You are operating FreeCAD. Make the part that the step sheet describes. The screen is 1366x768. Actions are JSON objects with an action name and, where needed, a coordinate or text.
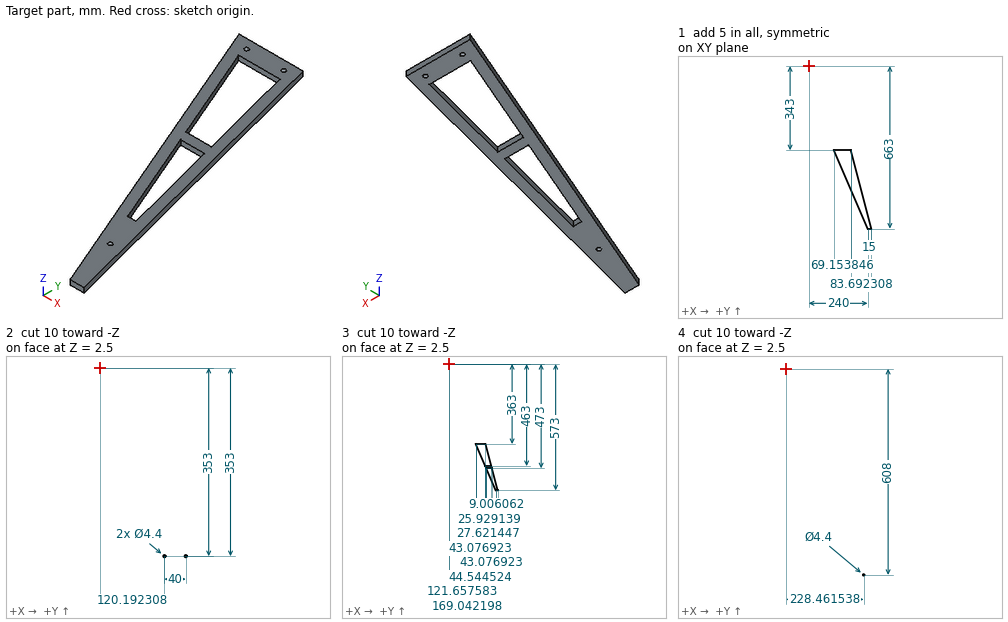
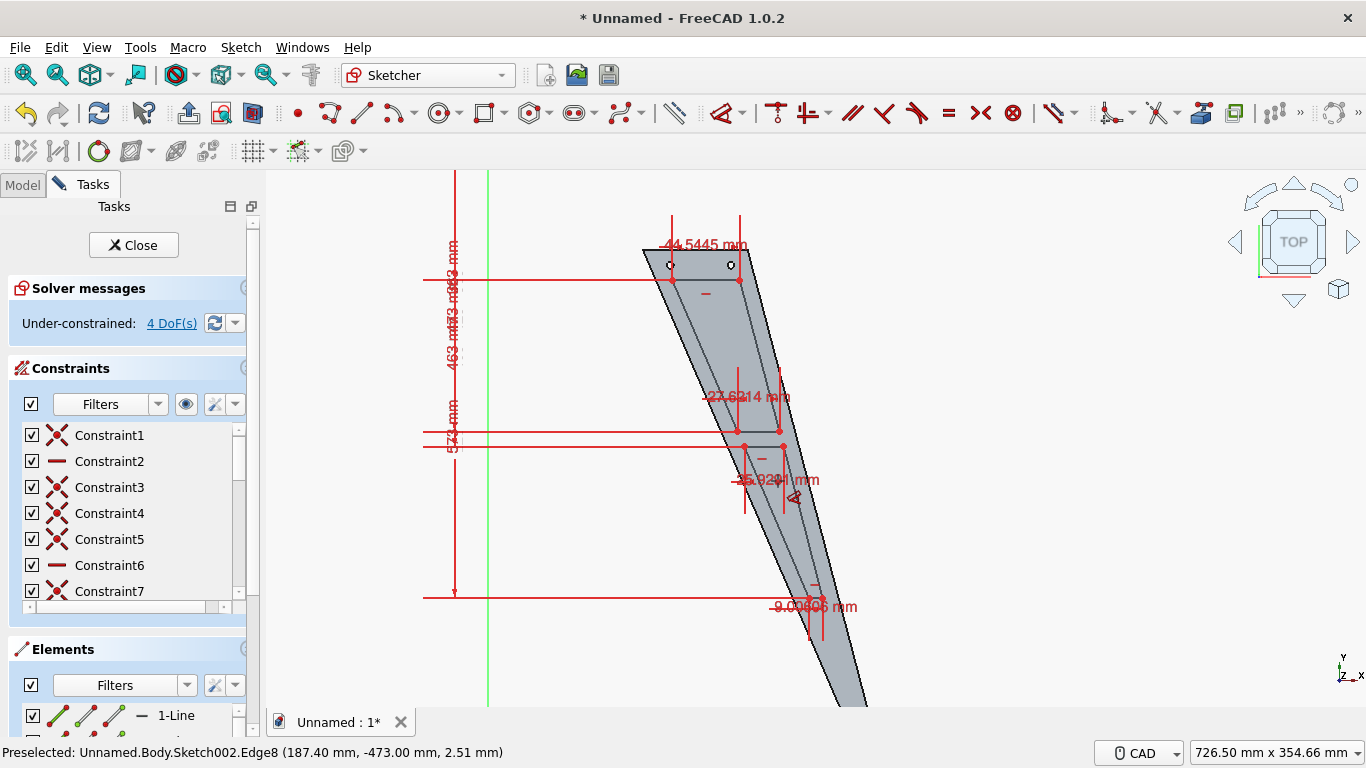
{"action": "left_click", "coordinate": [692, 326]}
{"action": "left_click", "coordinate": [705, 466]}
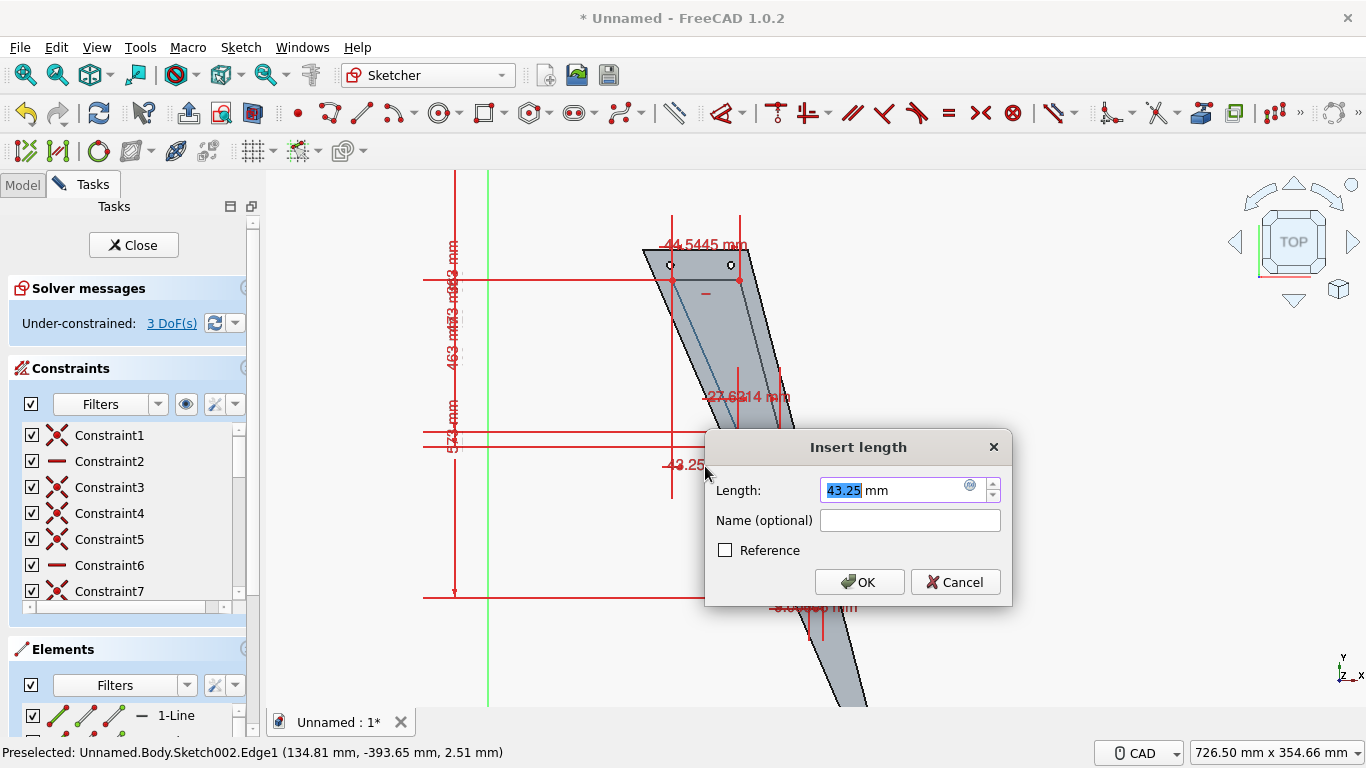
{"action": "type", "text": "43.076923"}
{"action": "key", "text": "Return"}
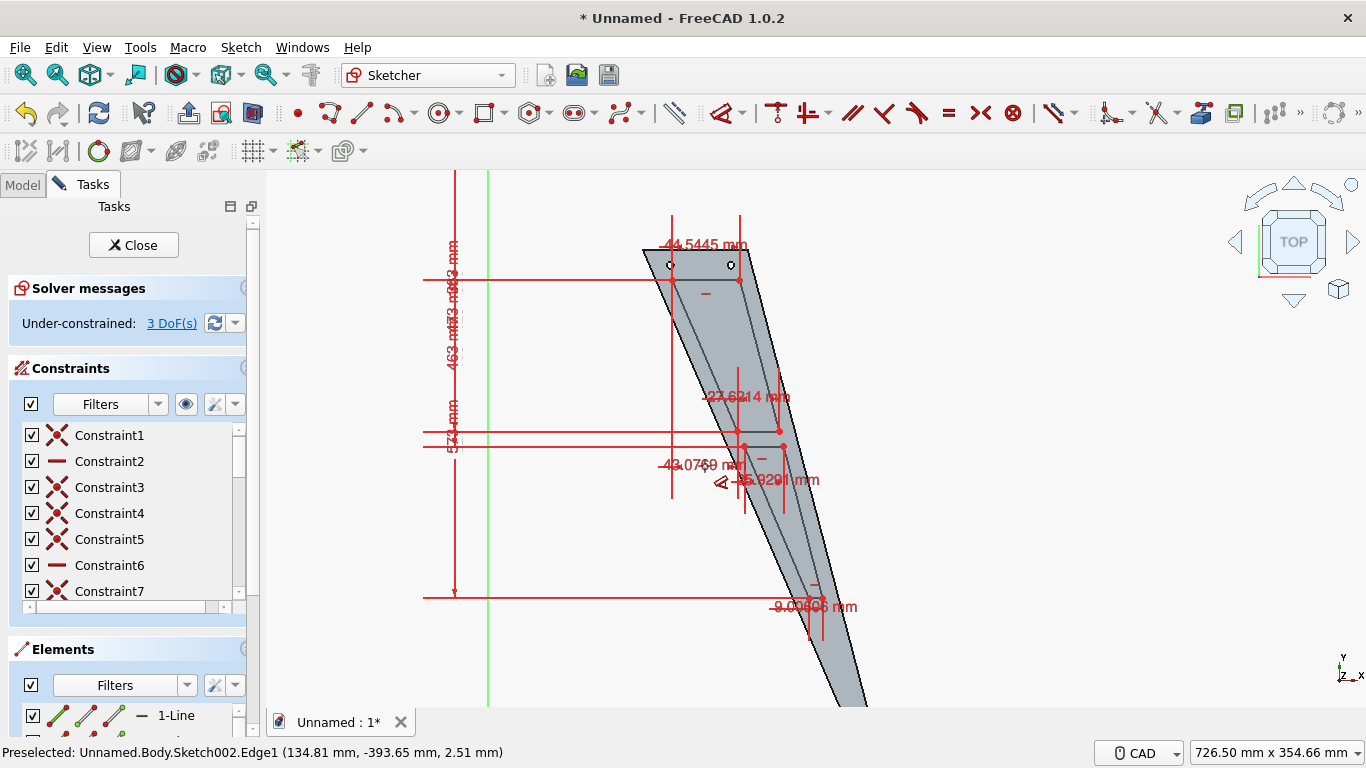
{"action": "left_click", "coordinate": [764, 492]}
{"action": "left_click", "coordinate": [777, 632]}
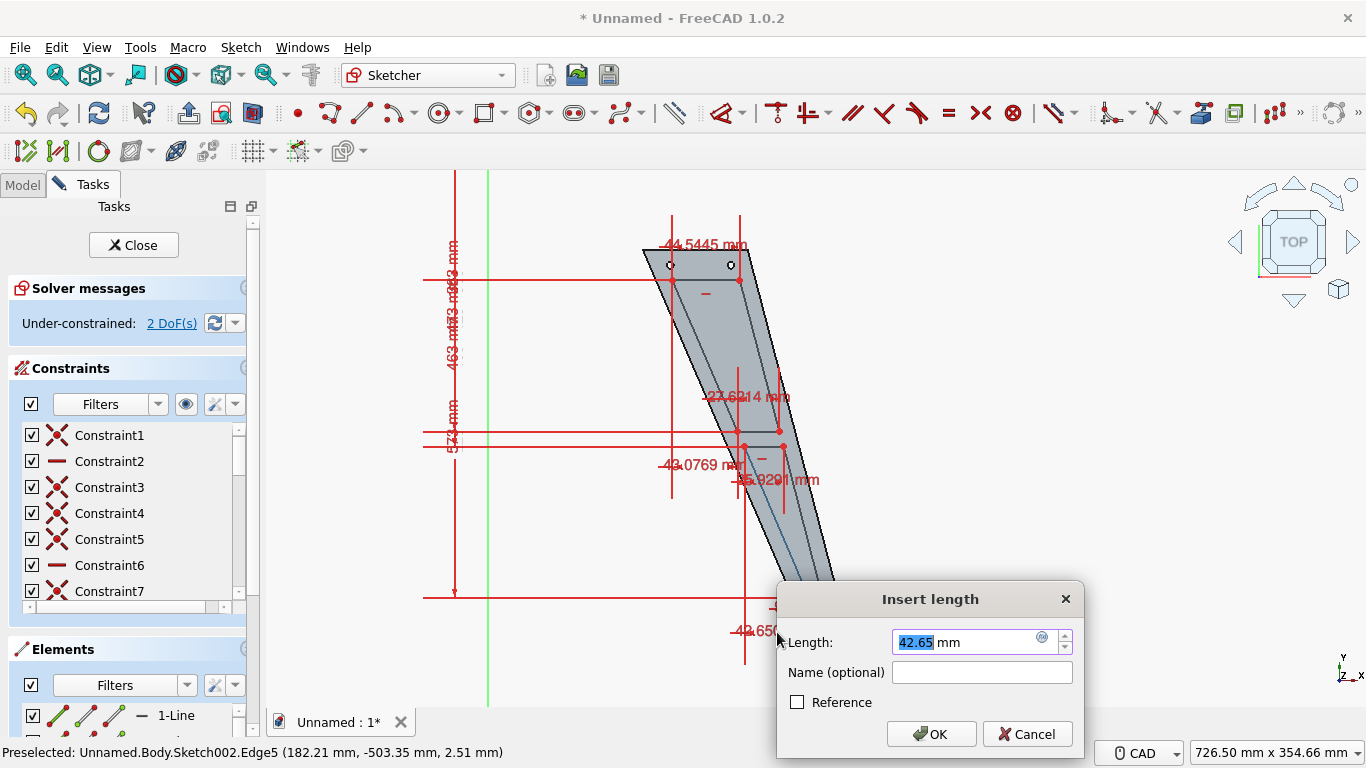
{"action": "type", "text": "43.076923"}
{"action": "key", "text": "Return"}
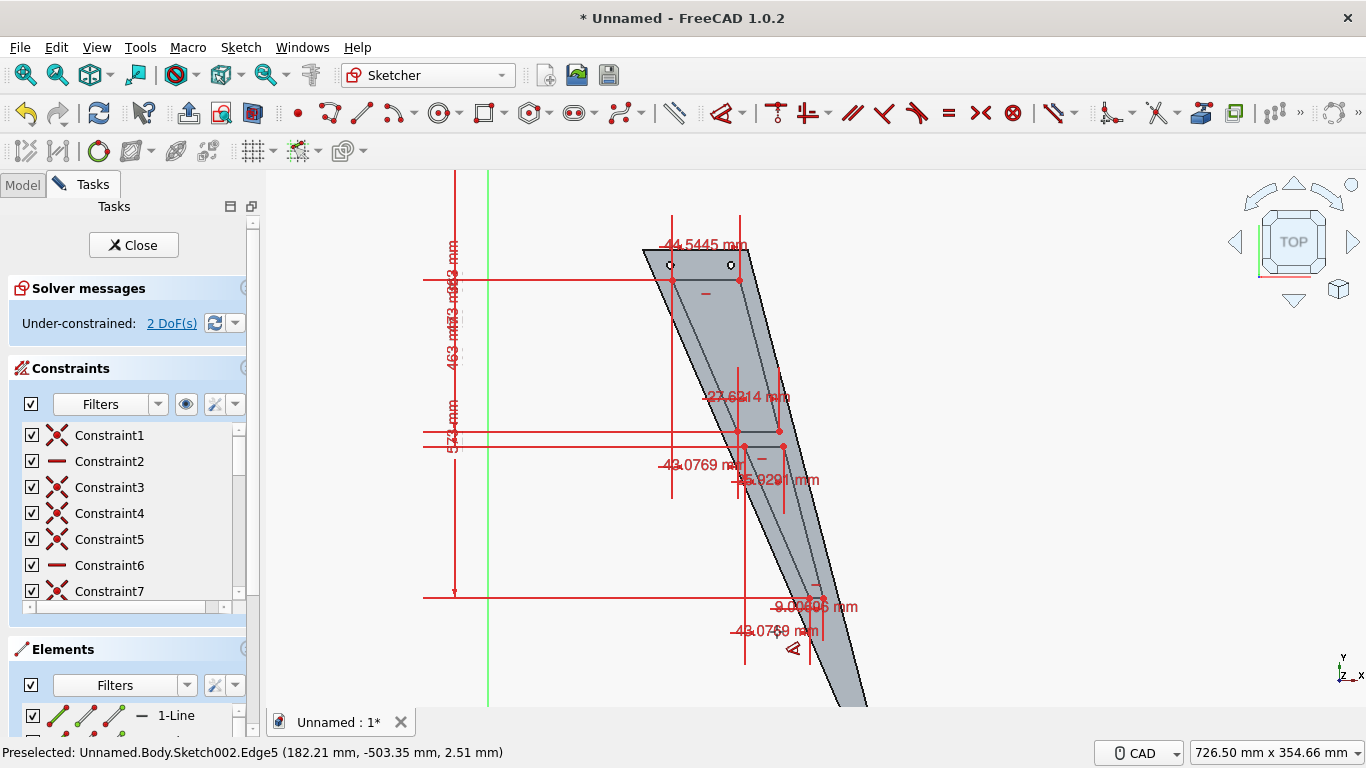
{"action": "left_click", "coordinate": [672, 280]}
{"action": "left_click", "coordinate": [580, 314]}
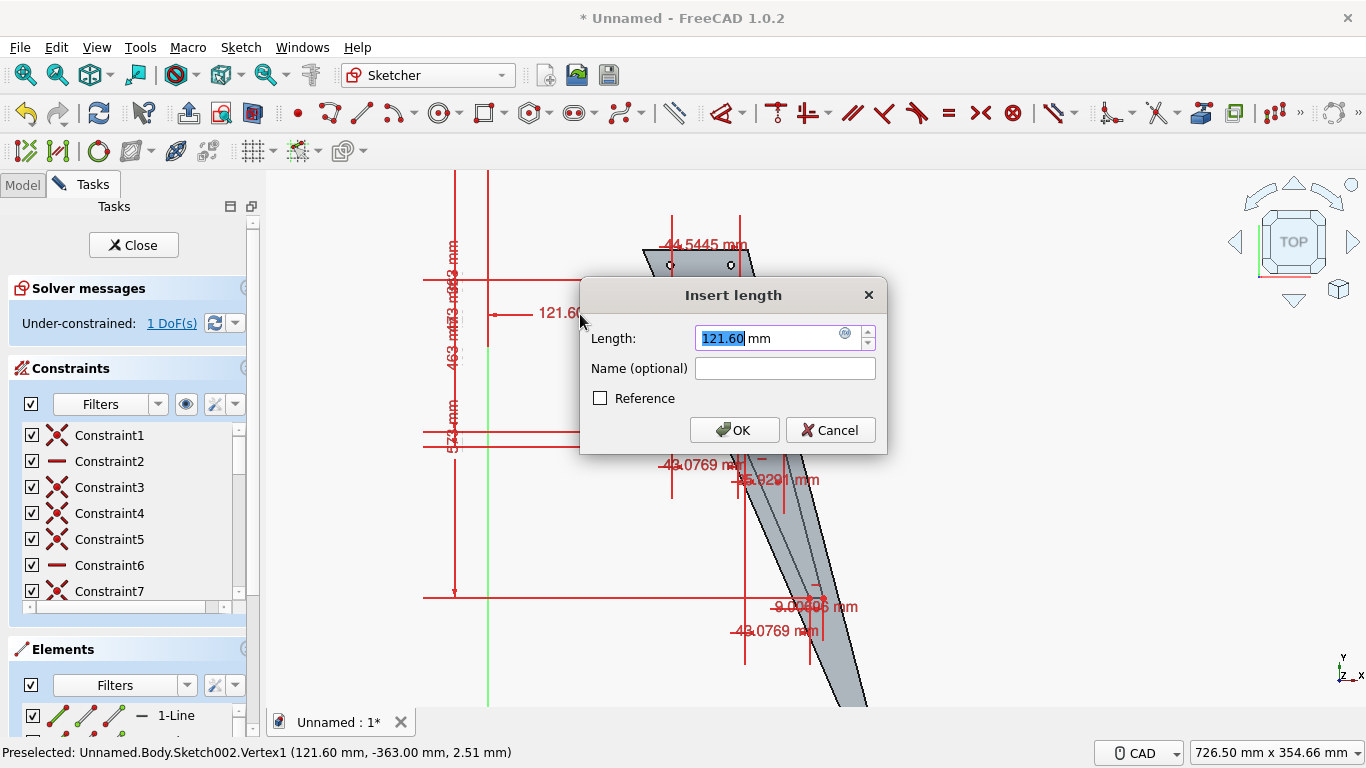
{"action": "type", "text": "121.657583"}
{"action": "key", "text": "Return"}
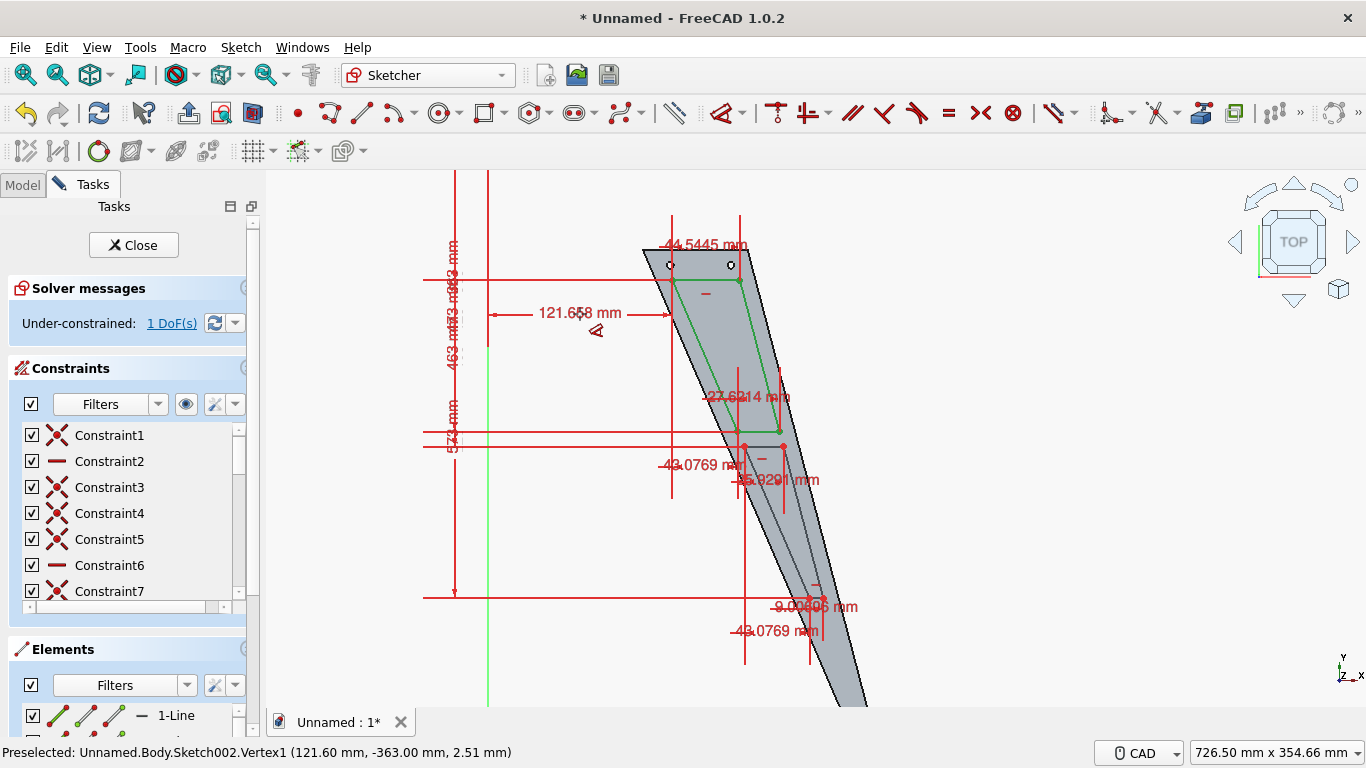
{"action": "left_click", "coordinate": [745, 447]}
{"action": "left_click", "coordinate": [616, 481]}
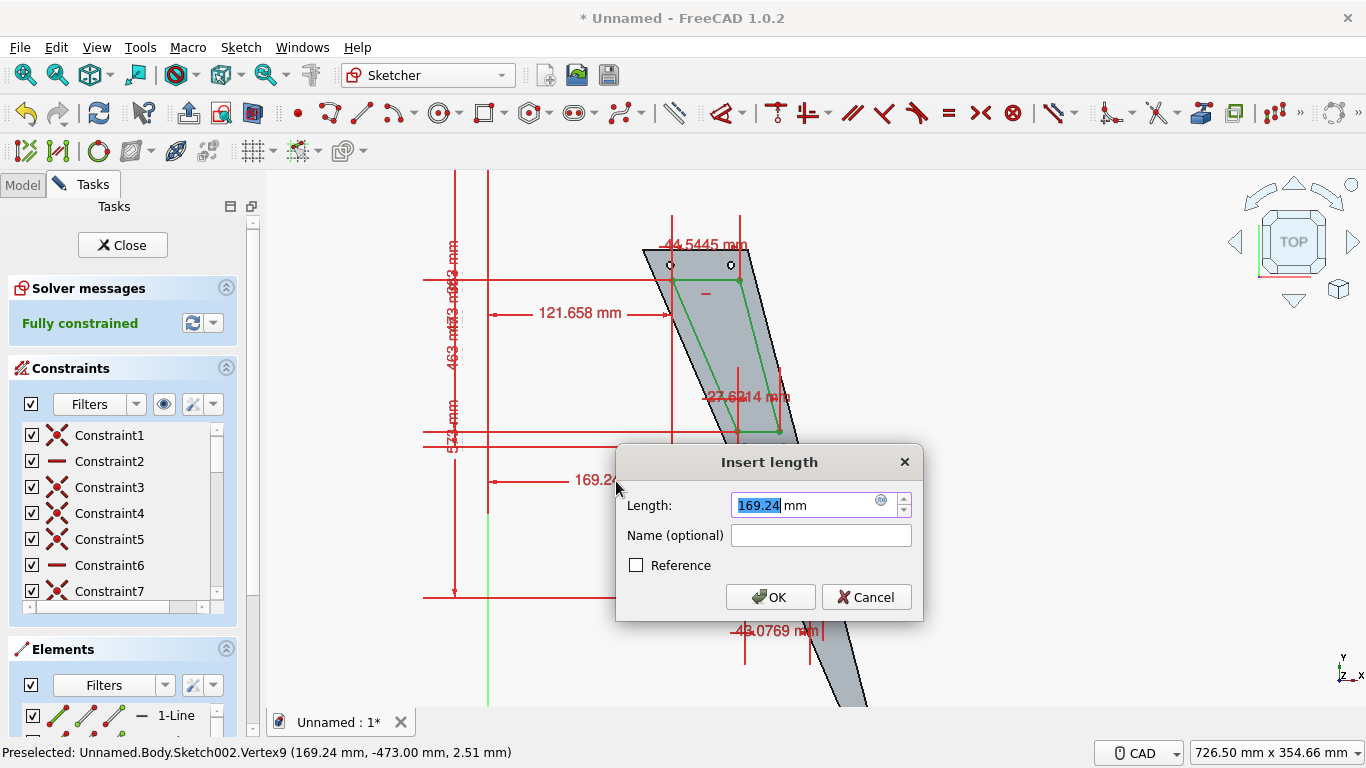
{"action": "type", "text": "169.042198"}
{"action": "key", "text": "Return"}
{"action": "key", "text": "Escape"}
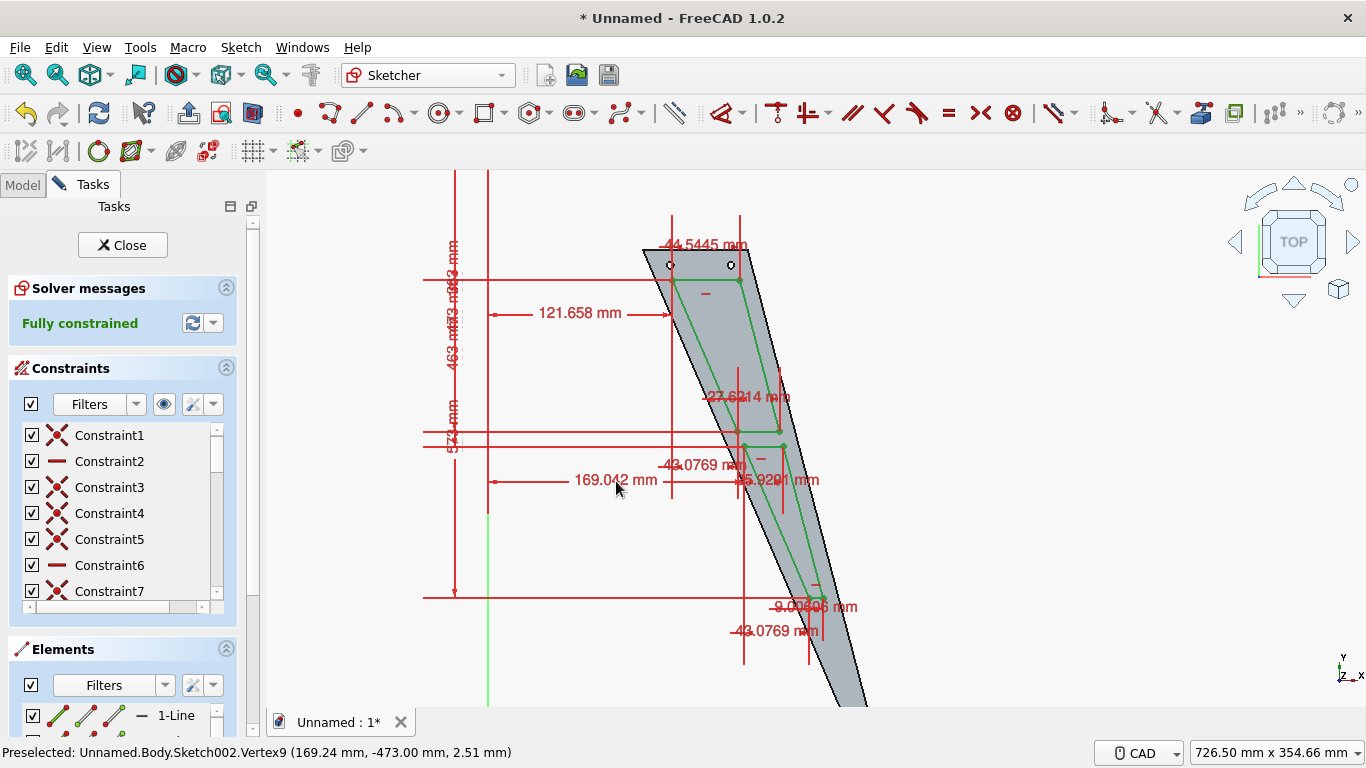
{"action": "left_click", "coordinate": [123, 245]}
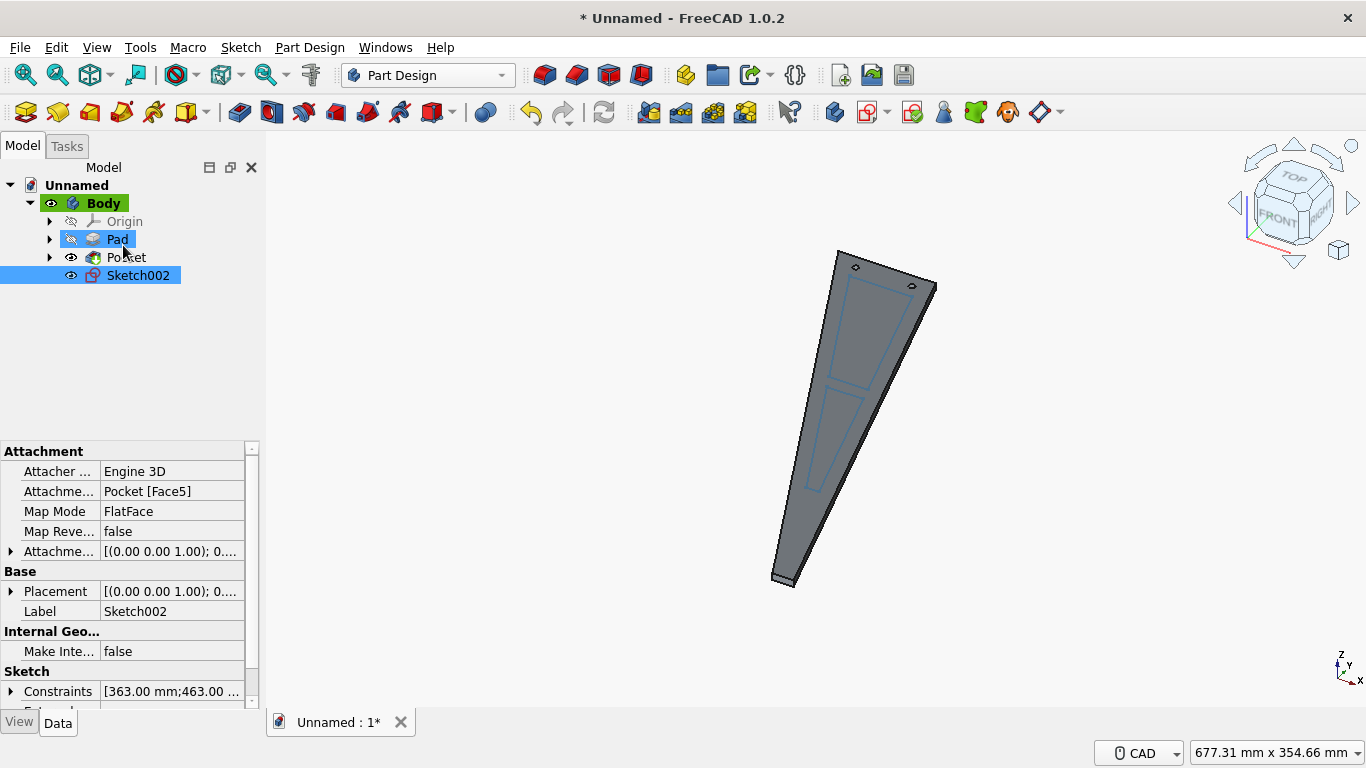
{"action": "left_click", "coordinate": [240, 112]}